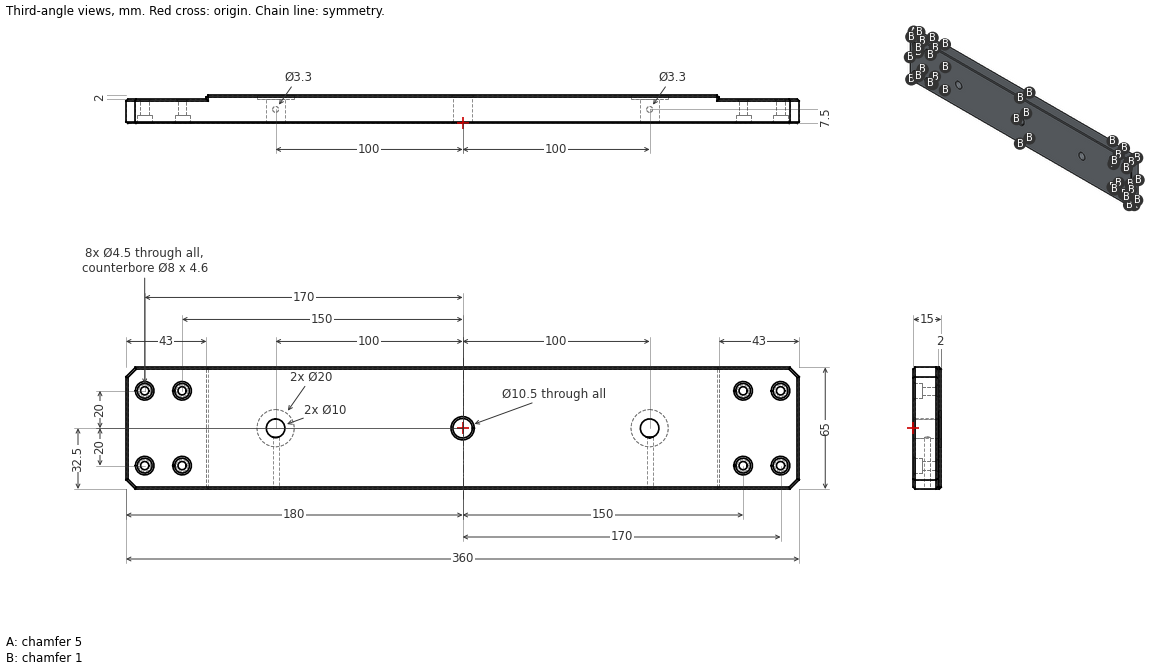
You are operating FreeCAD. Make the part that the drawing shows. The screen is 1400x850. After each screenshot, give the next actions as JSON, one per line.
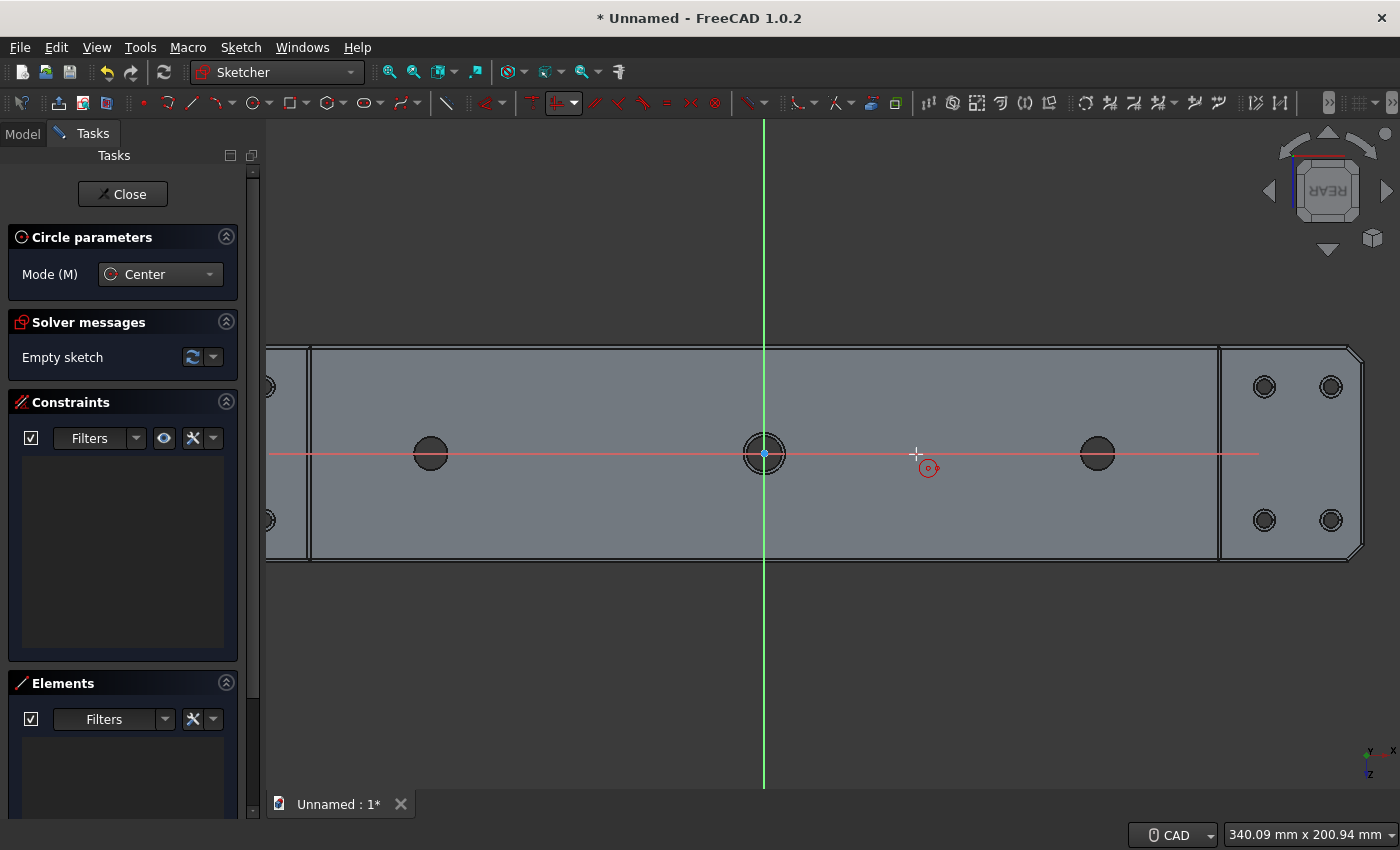
{"action": "left_click", "coordinate": [431, 454]}
{"action": "mouse_move", "coordinate": [454, 430]}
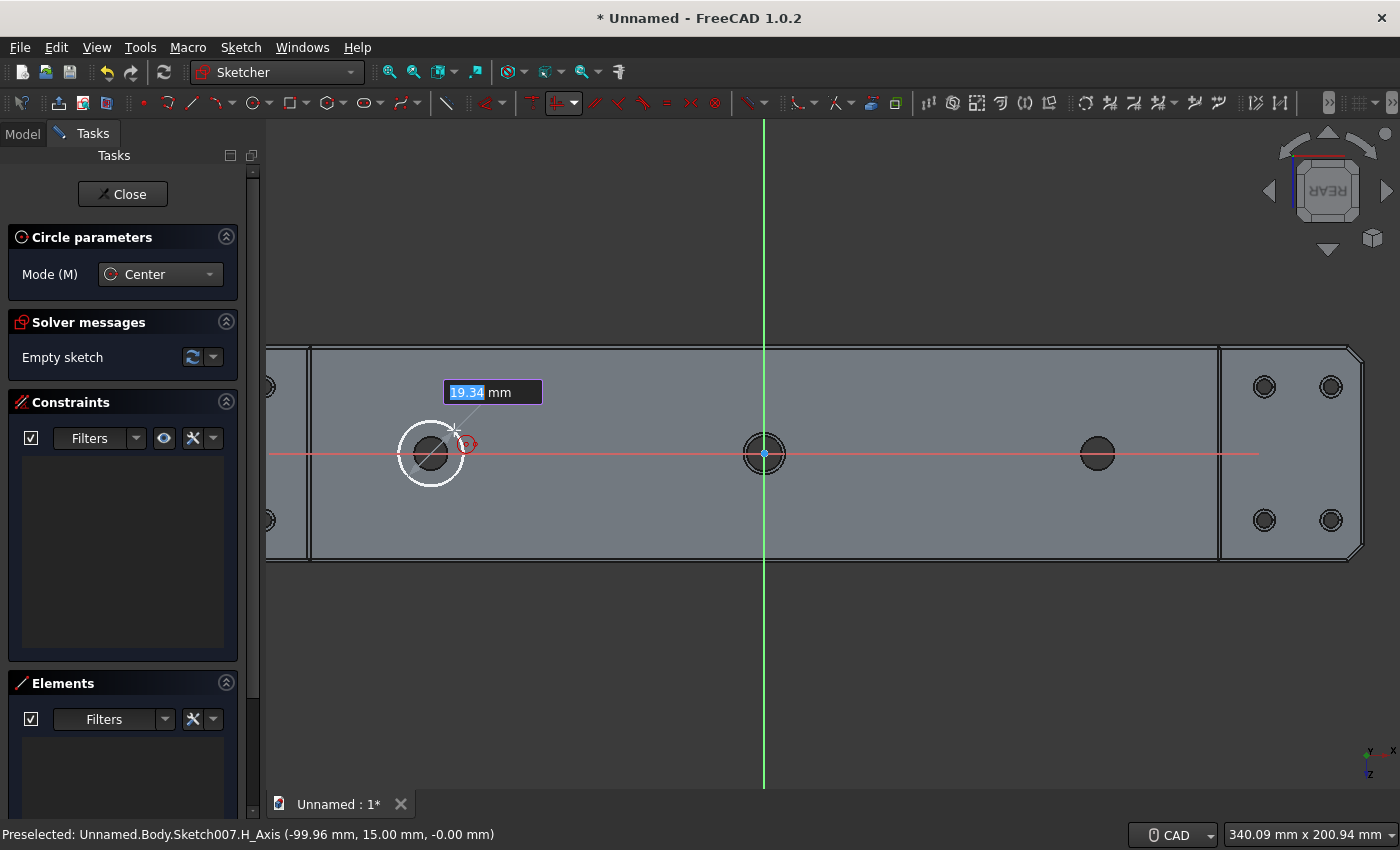
{"action": "type", "text": "20"}
{"action": "key", "text": "Return"}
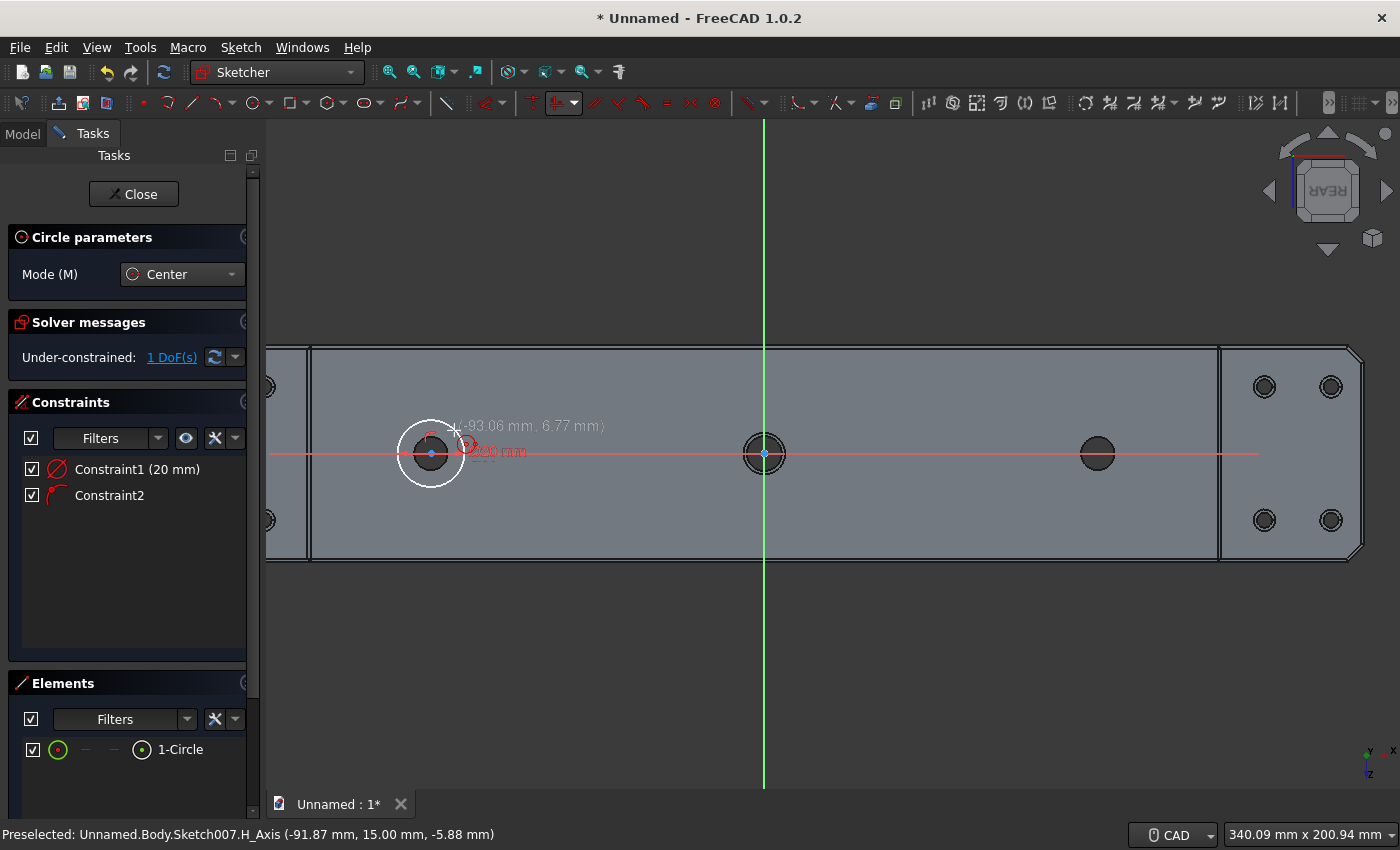
{"action": "left_click", "coordinate": [1098, 454]}
{"action": "mouse_move", "coordinate": [1121, 430]}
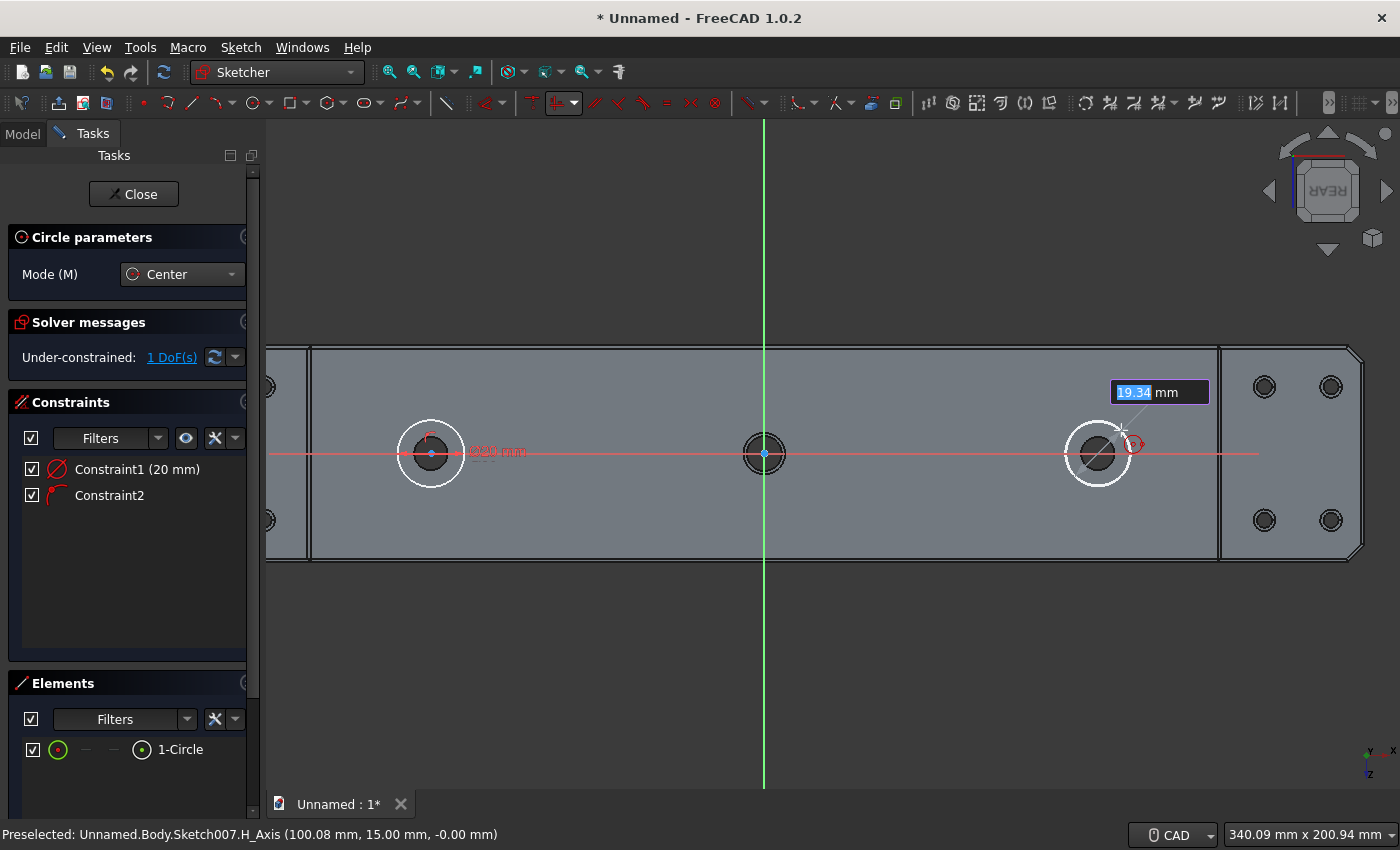
{"action": "type", "text": "20"}
{"action": "key", "text": "Return"}
{"action": "key", "text": "Escape"}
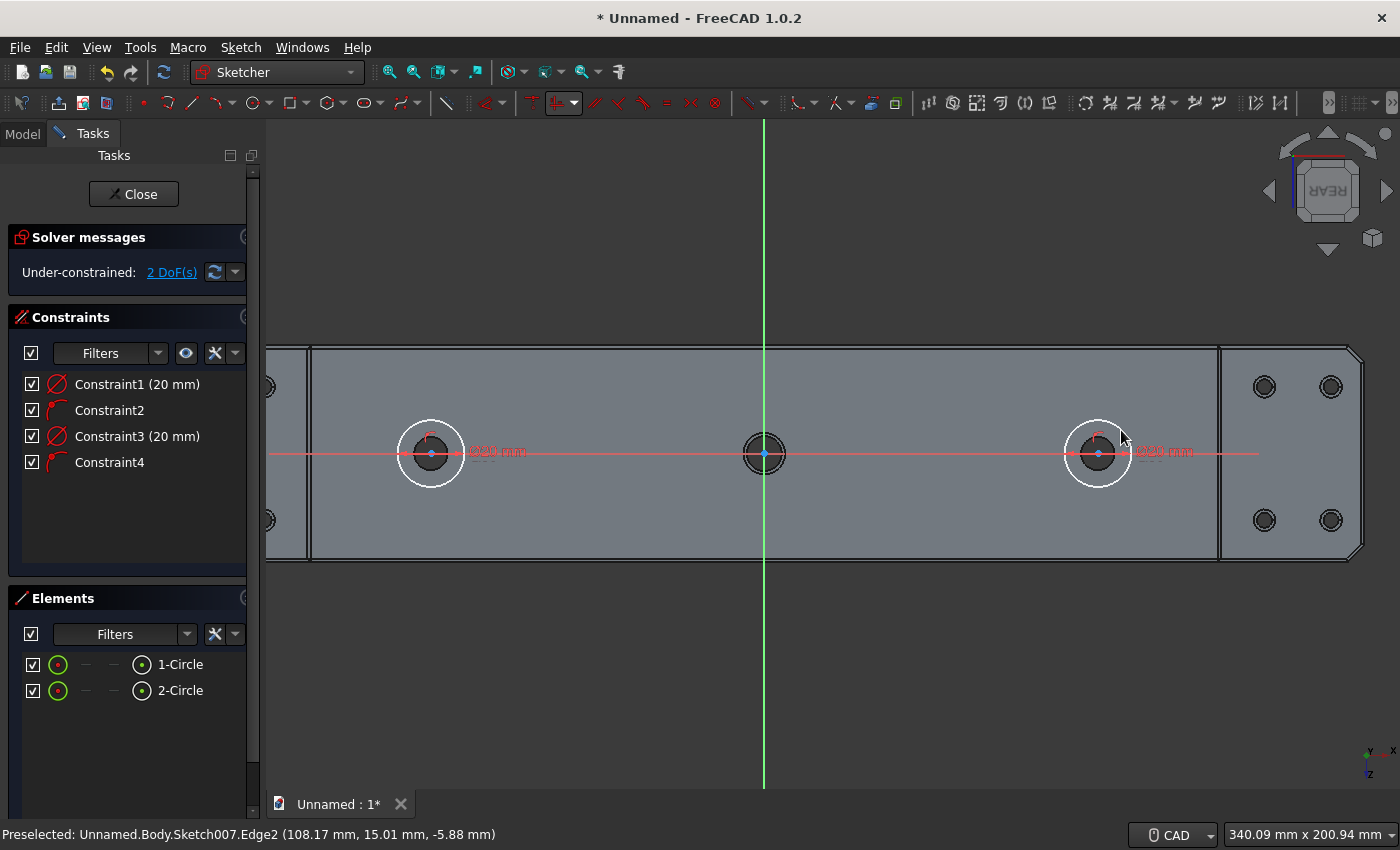
{"action": "left_click", "coordinate": [486, 104]}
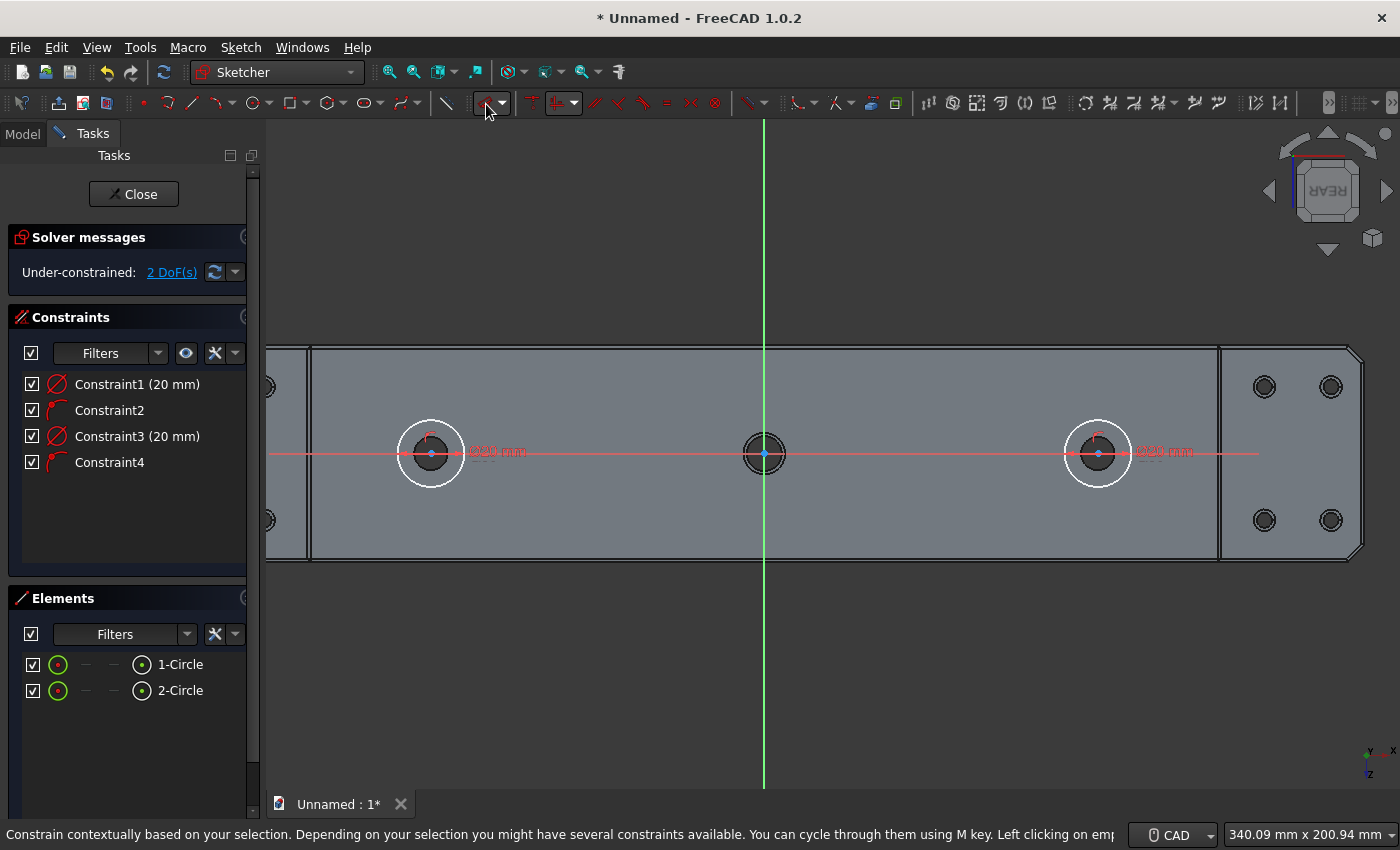
{"action": "left_click", "coordinate": [431, 454]}
{"action": "left_click", "coordinate": [598, 488]}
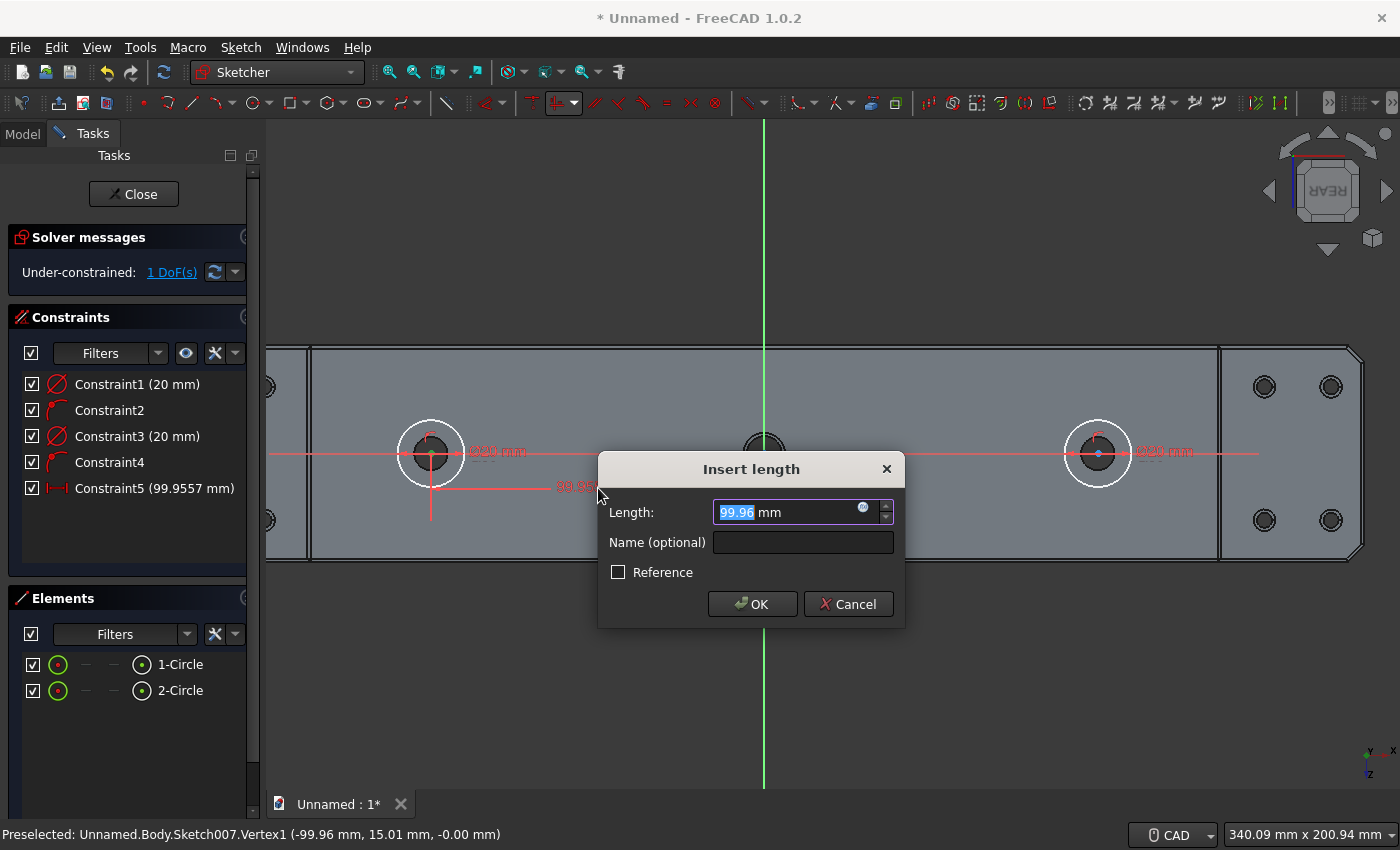
{"action": "type", "text": "100"}
{"action": "key", "text": "Return"}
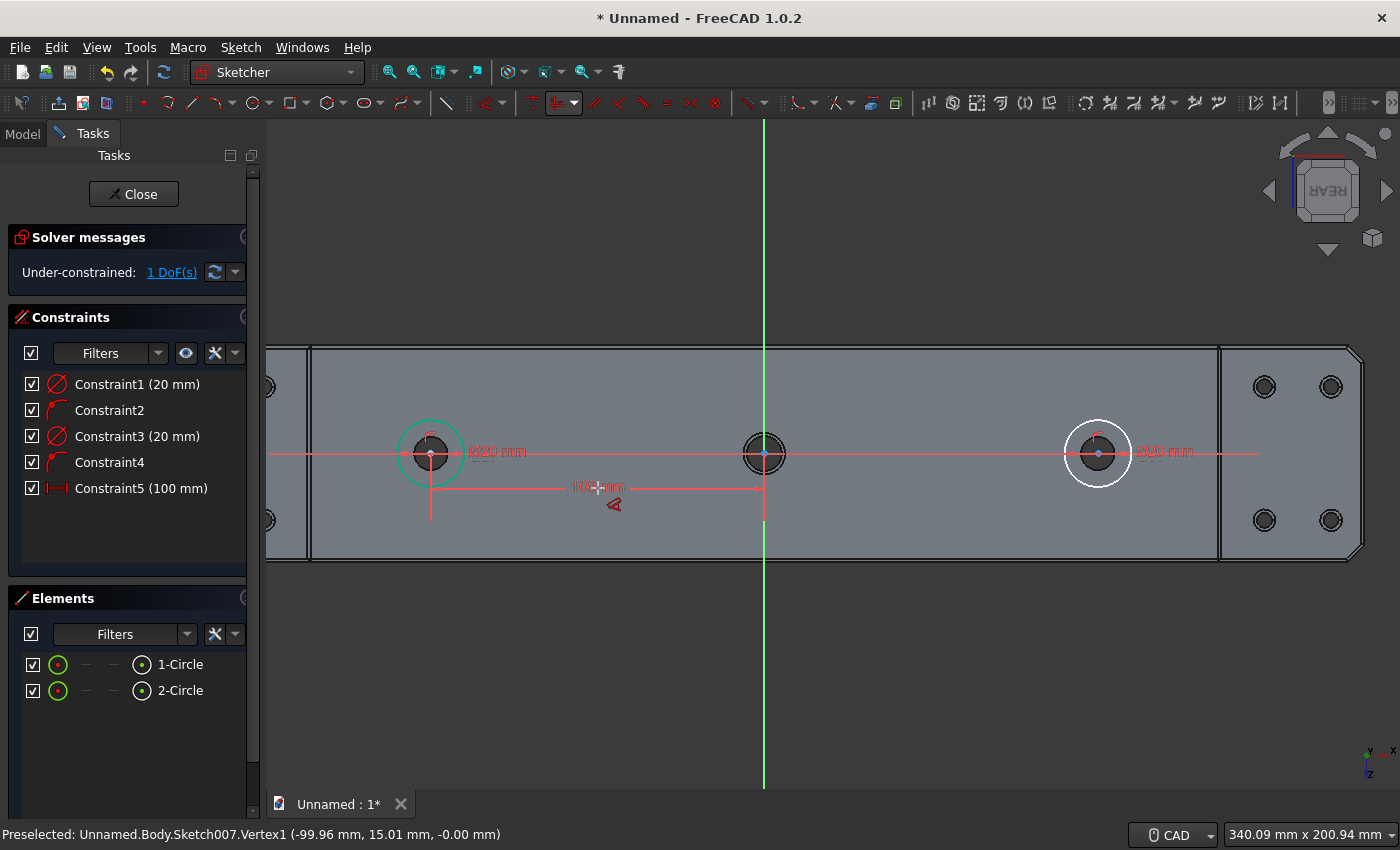
{"action": "left_click", "coordinate": [1098, 454]}
{"action": "left_click", "coordinate": [931, 488]}